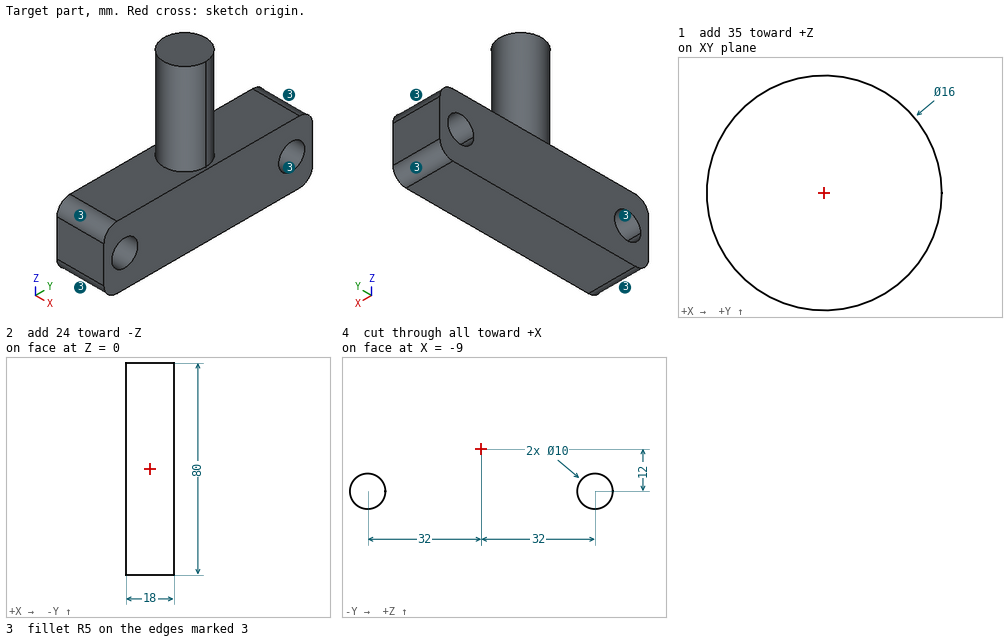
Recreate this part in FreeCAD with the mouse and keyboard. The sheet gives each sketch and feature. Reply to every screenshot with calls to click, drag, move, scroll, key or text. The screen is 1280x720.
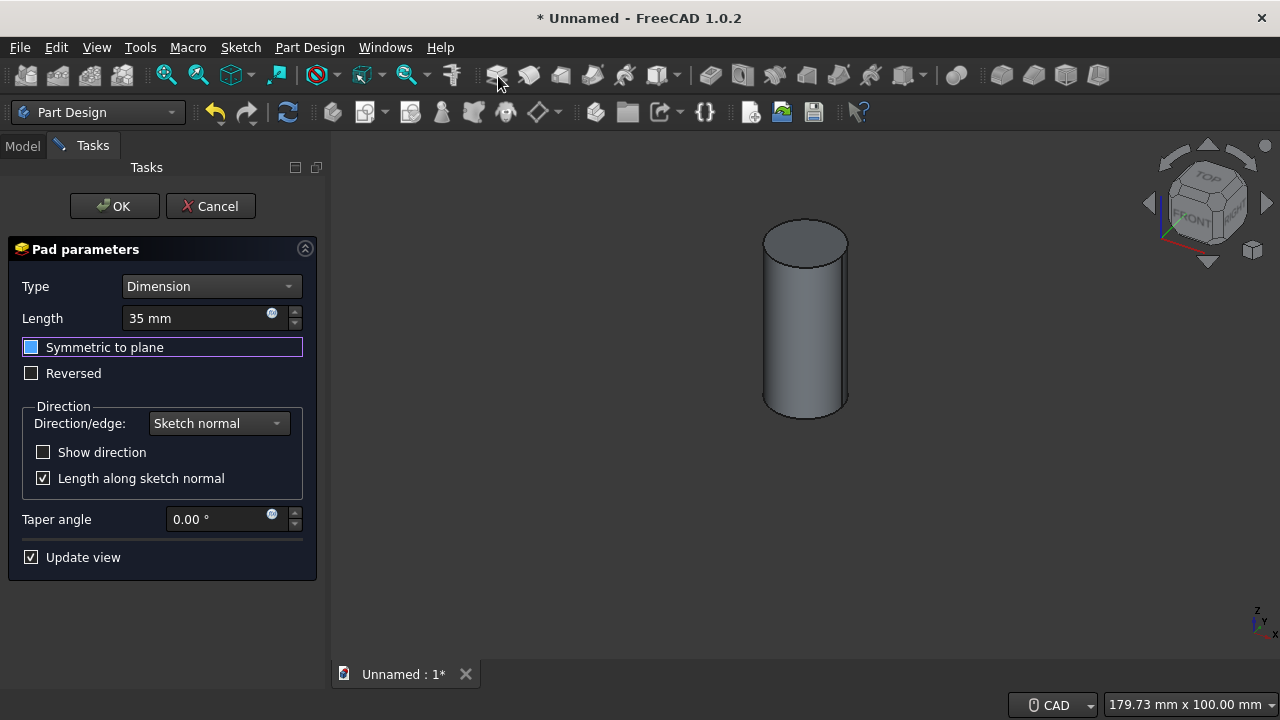
click(115, 206)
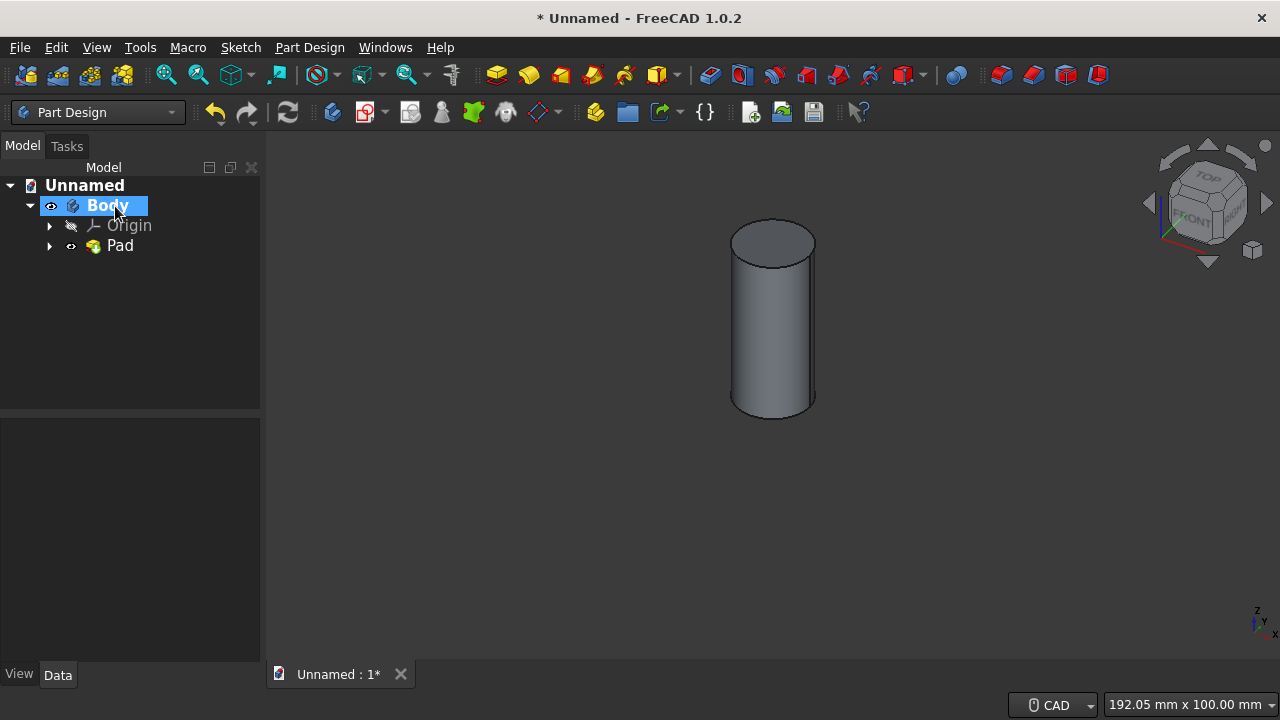
click(168, 76)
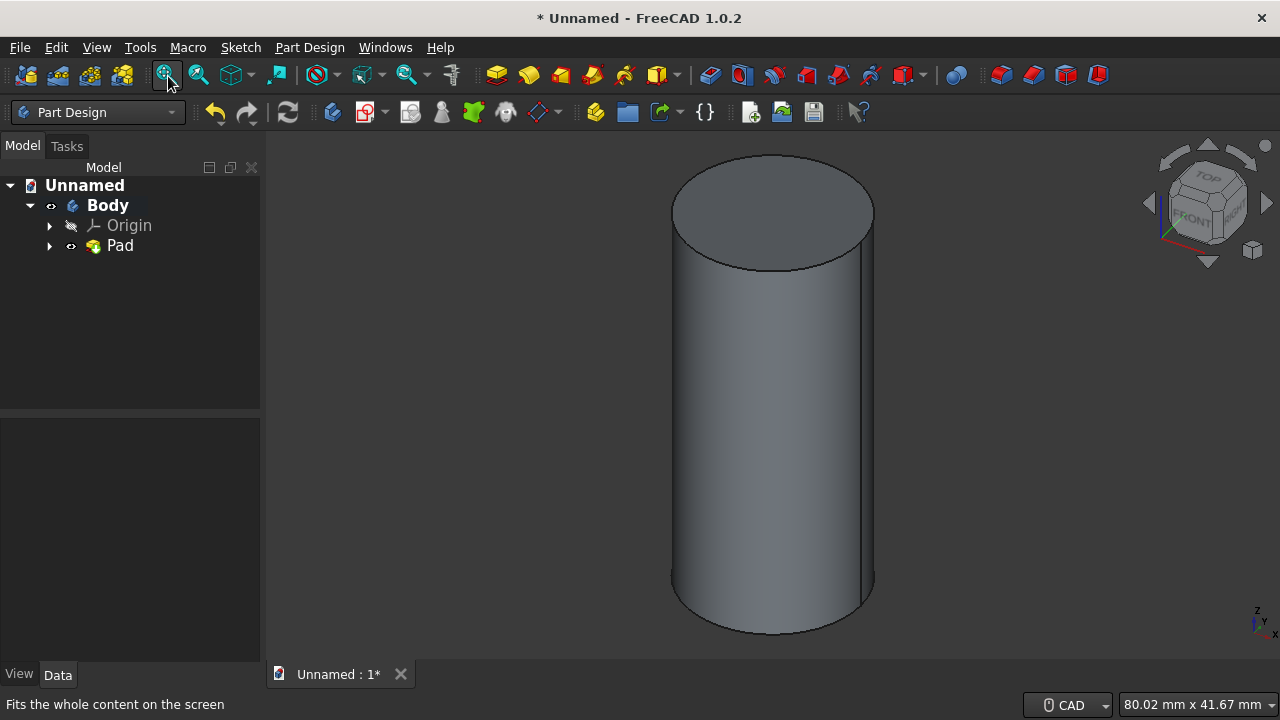
key(5)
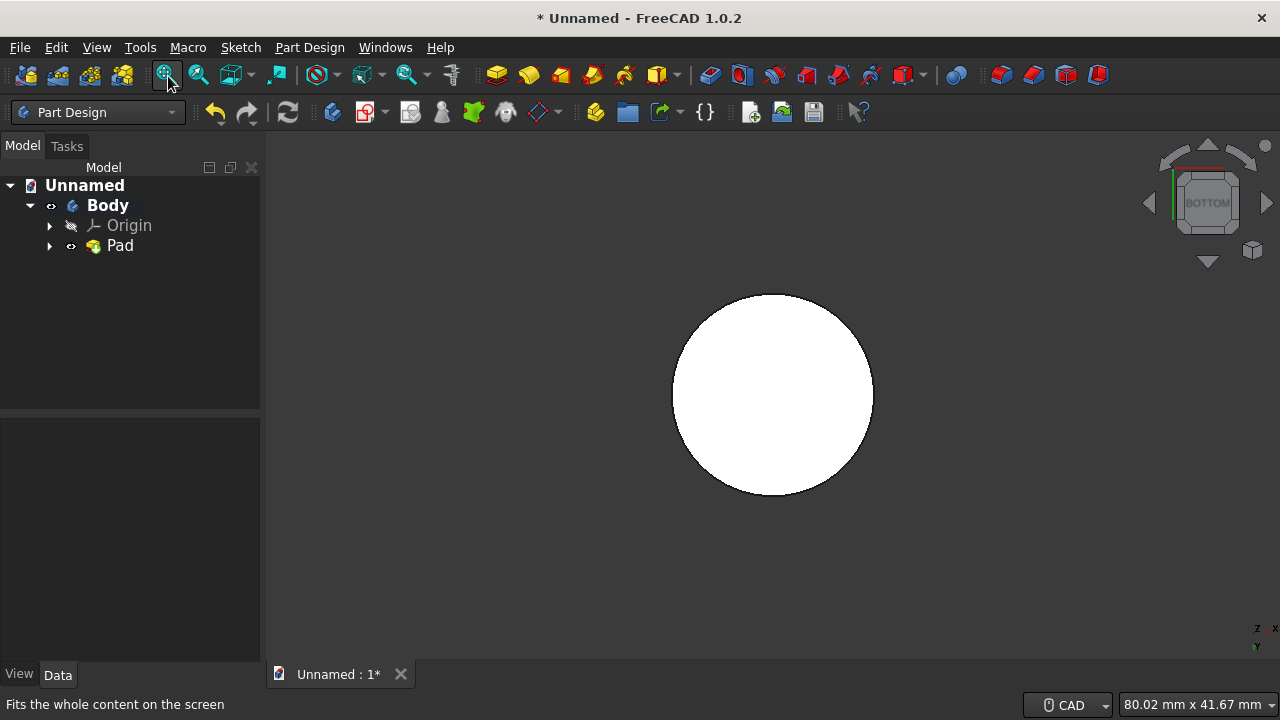
click(168, 76)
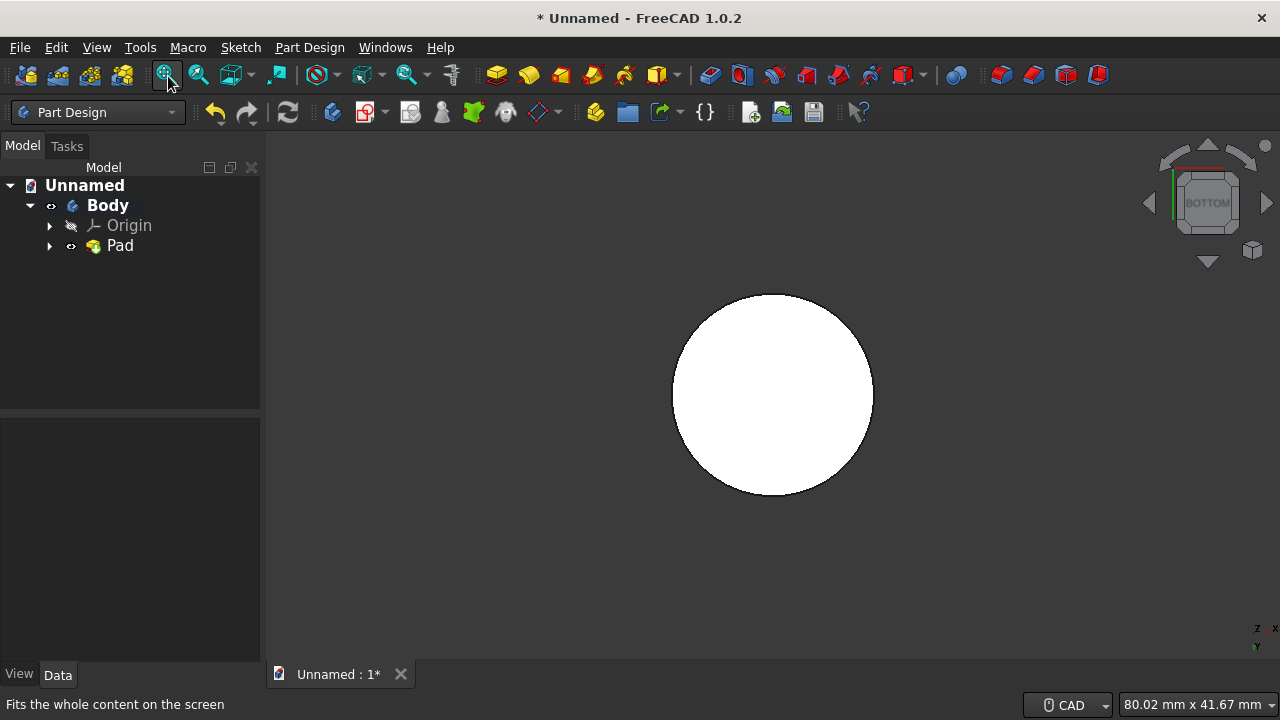
click(773, 394)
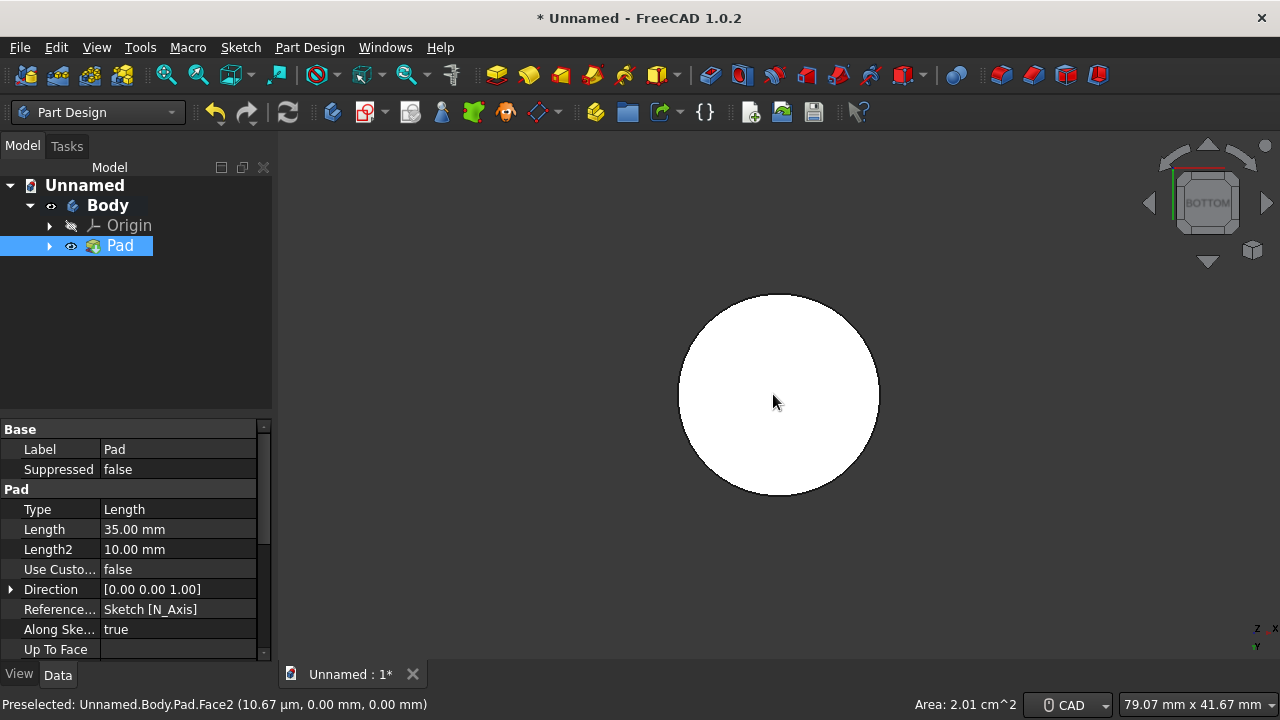
click(366, 112)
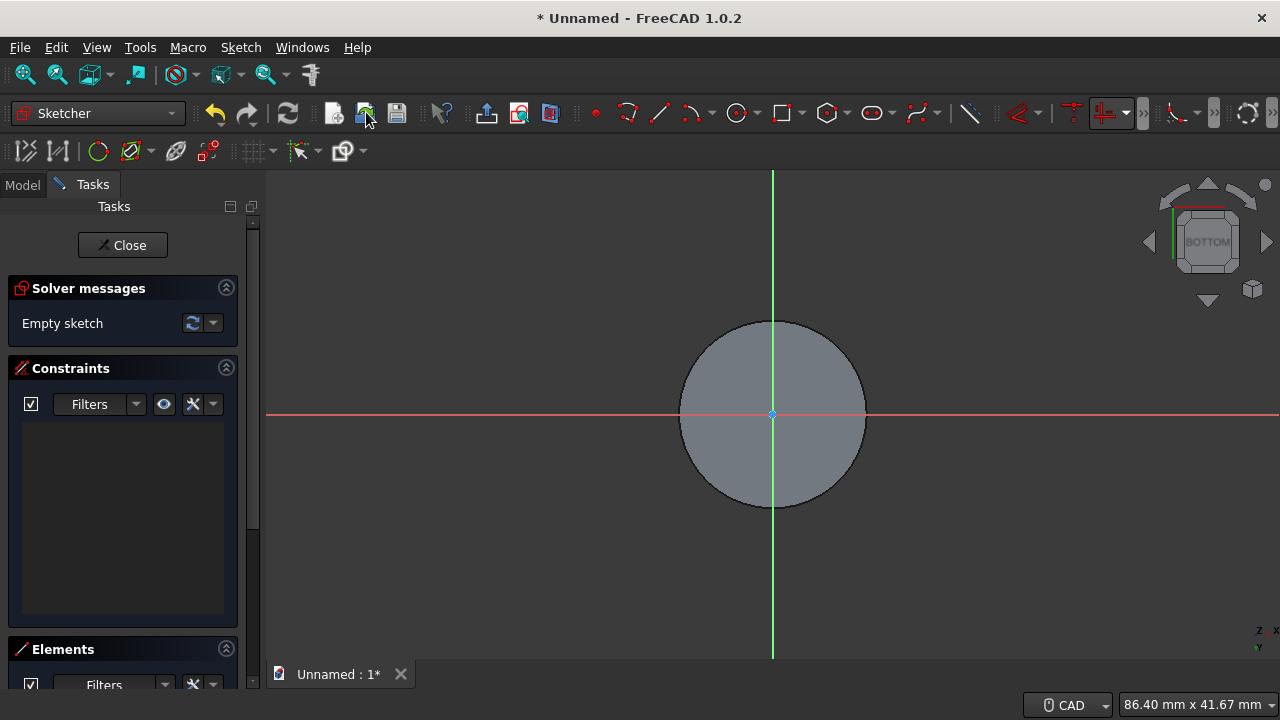
scroll(675, 414, down, 6)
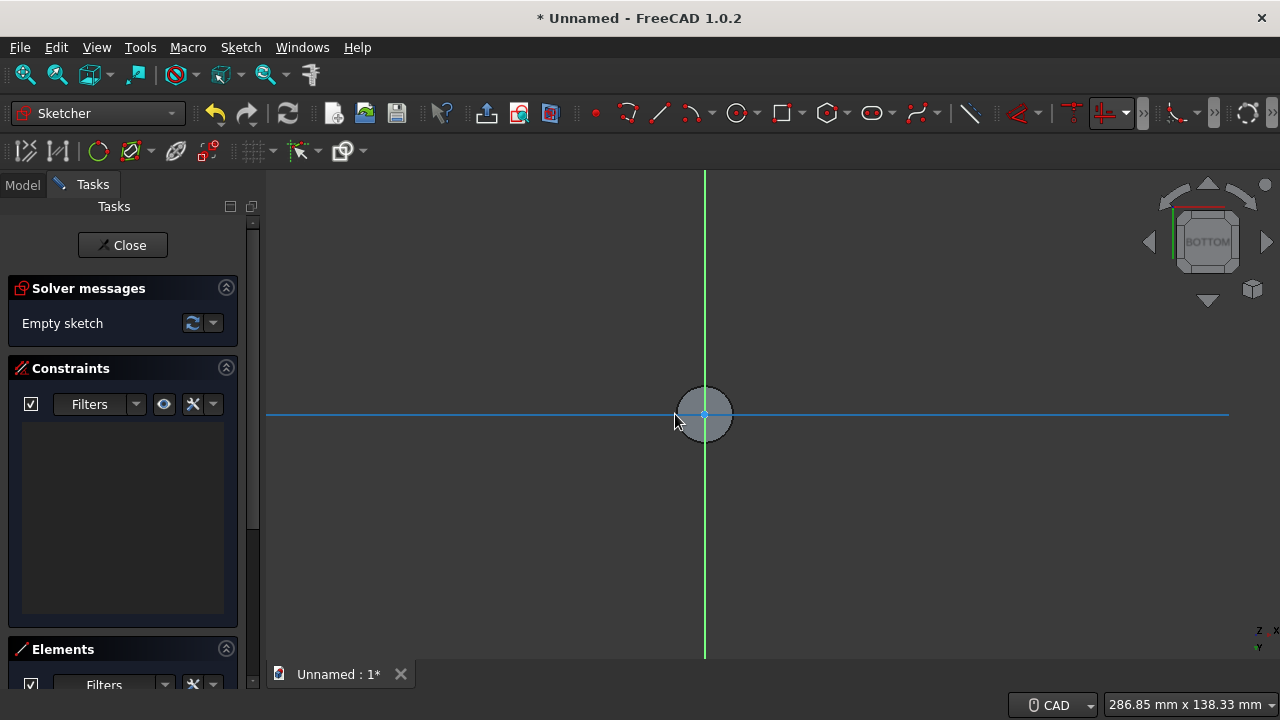
key(g)
key(v)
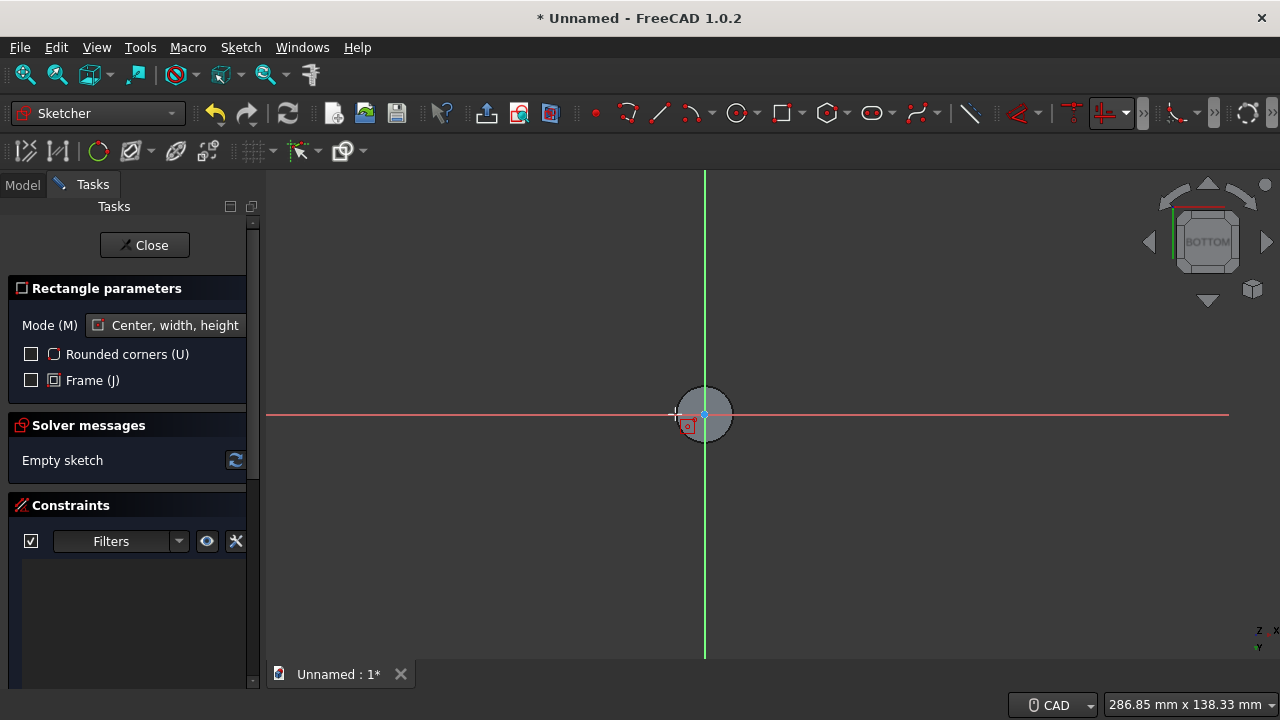
click(705, 414)
move(737, 273)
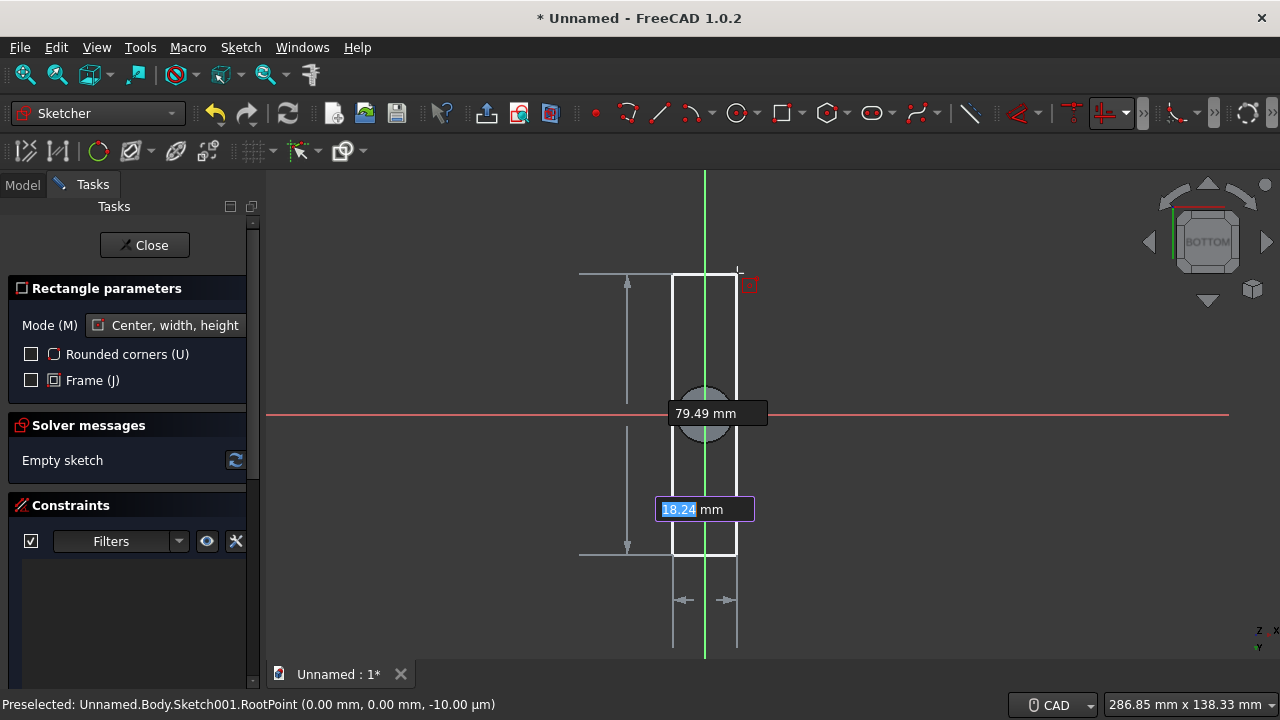
text(18)
key(Tab)
text(80)
key(Return)
key(Escape)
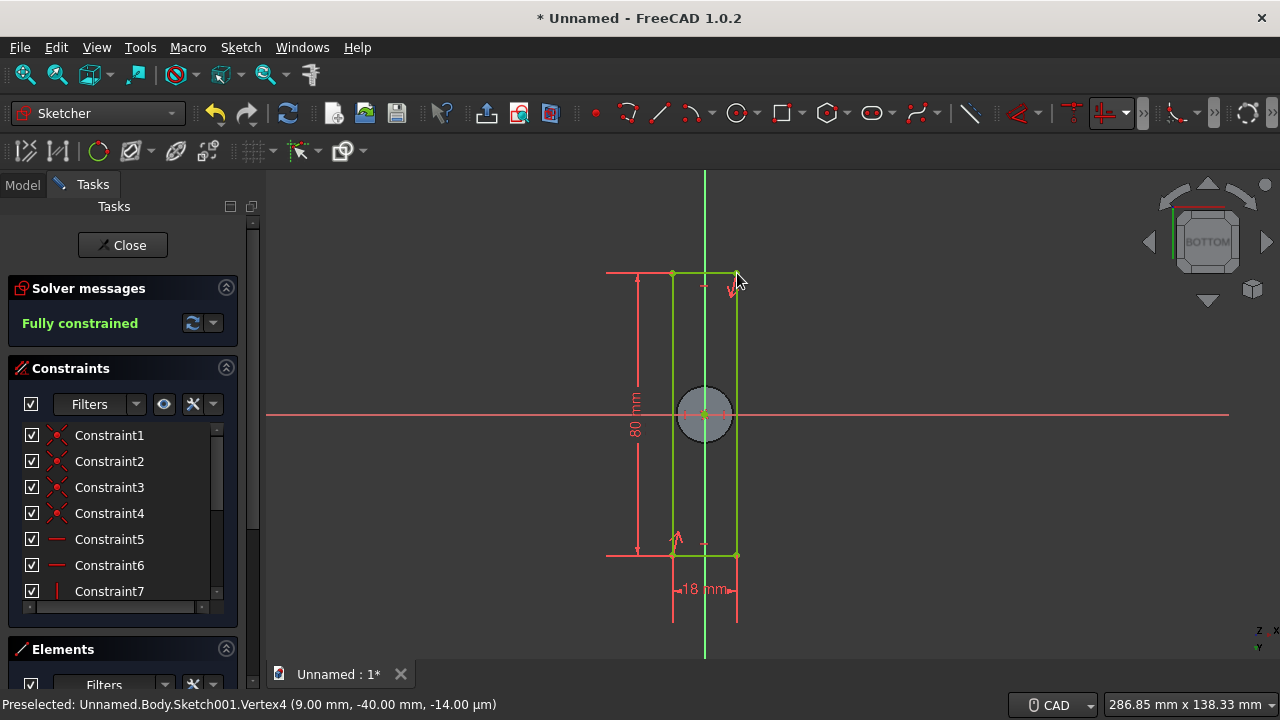
click(123, 245)